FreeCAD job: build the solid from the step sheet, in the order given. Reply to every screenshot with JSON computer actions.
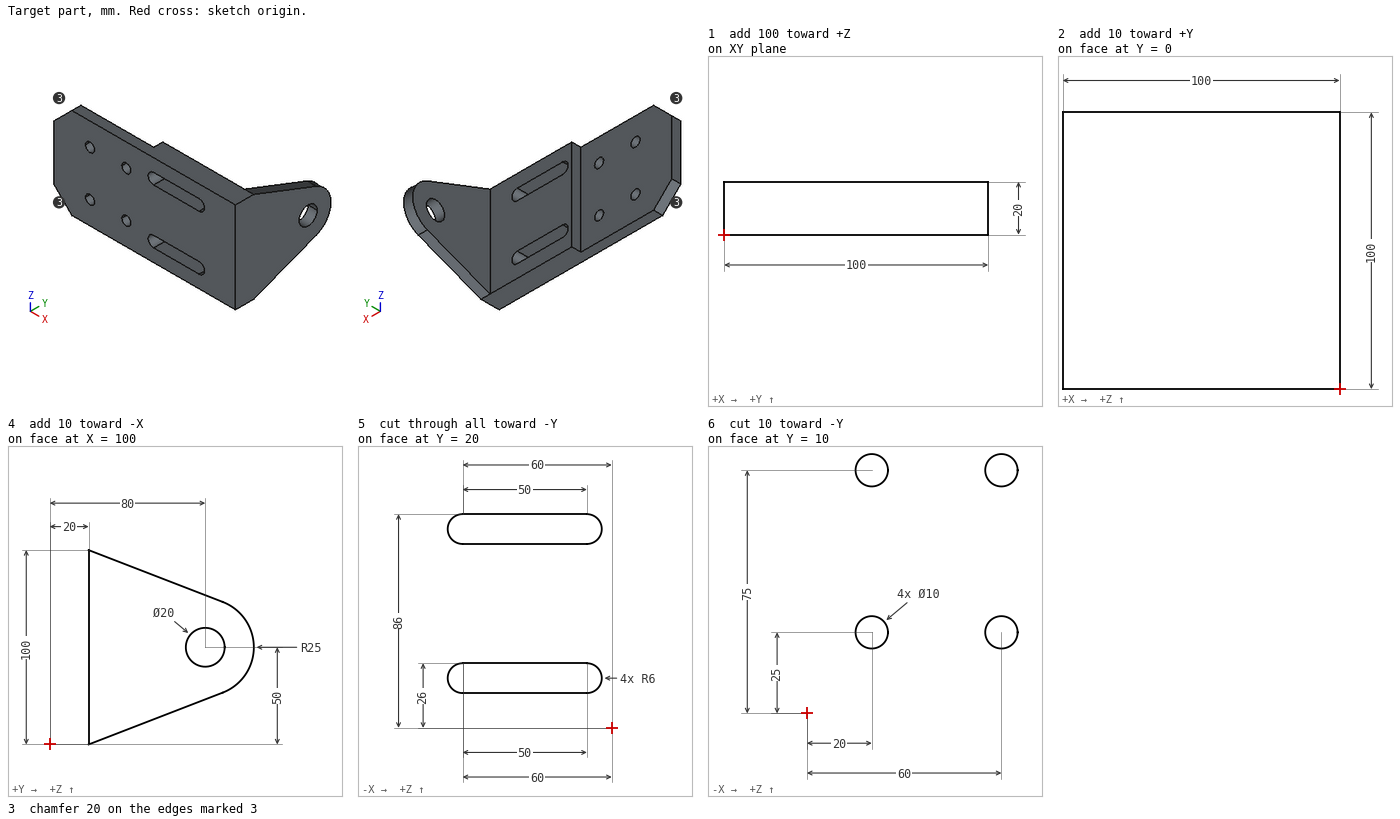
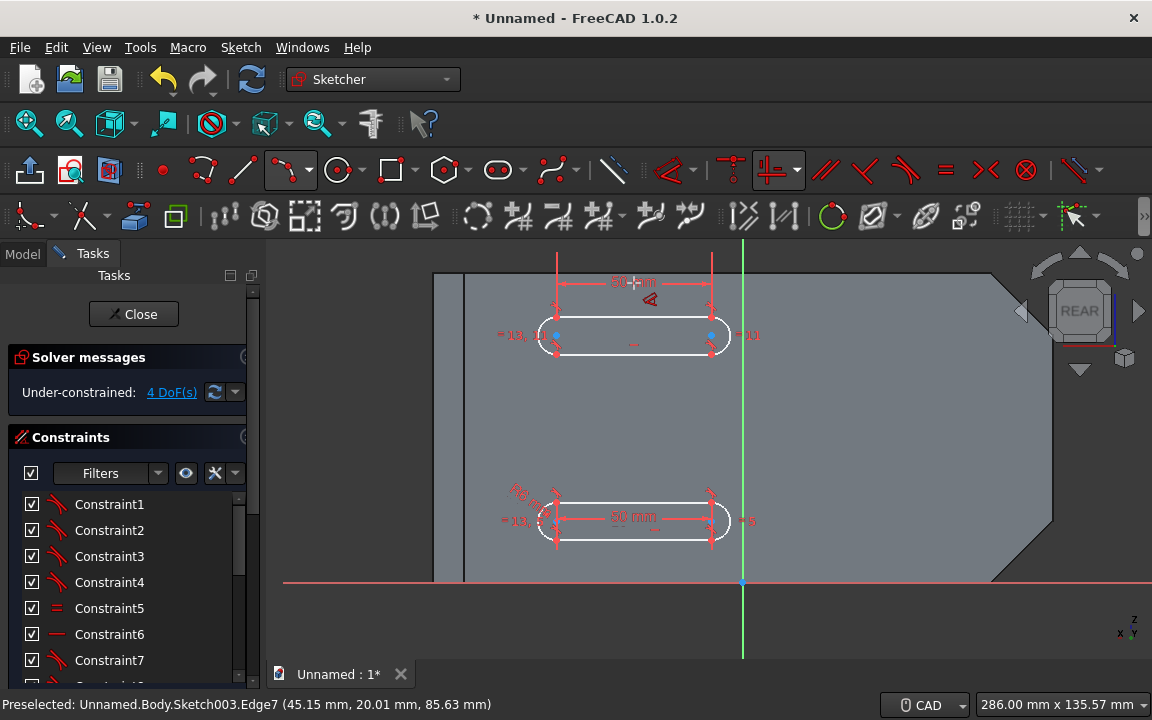
{"action": "left_click", "coordinate": [557, 503]}
{"action": "left_click", "coordinate": [650, 617]}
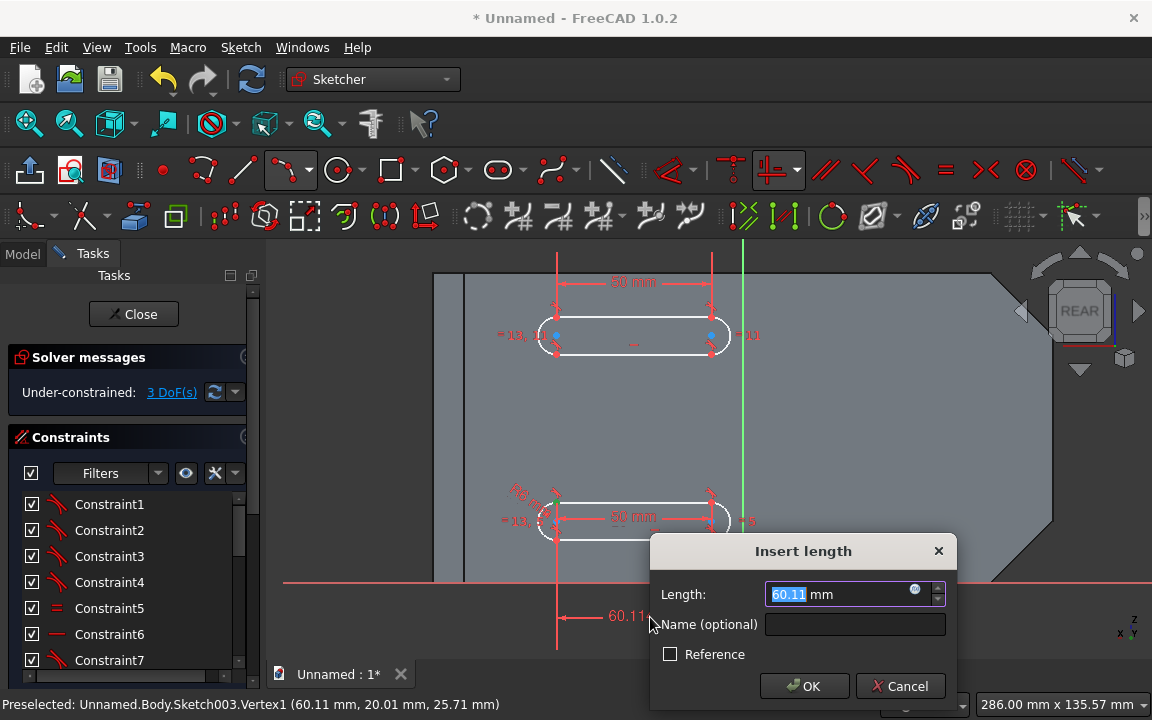
{"action": "type", "text": "60"}
{"action": "key", "text": "Return"}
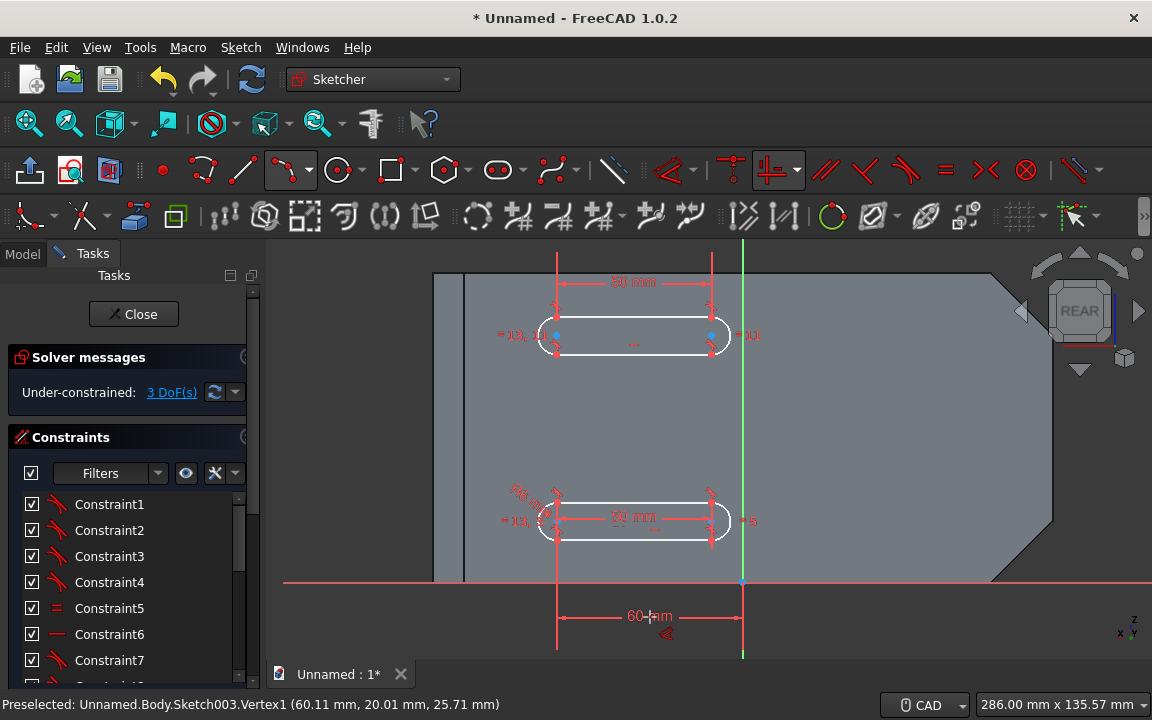
{"action": "left_click", "coordinate": [557, 503]}
{"action": "left_click", "coordinate": [777, 543]}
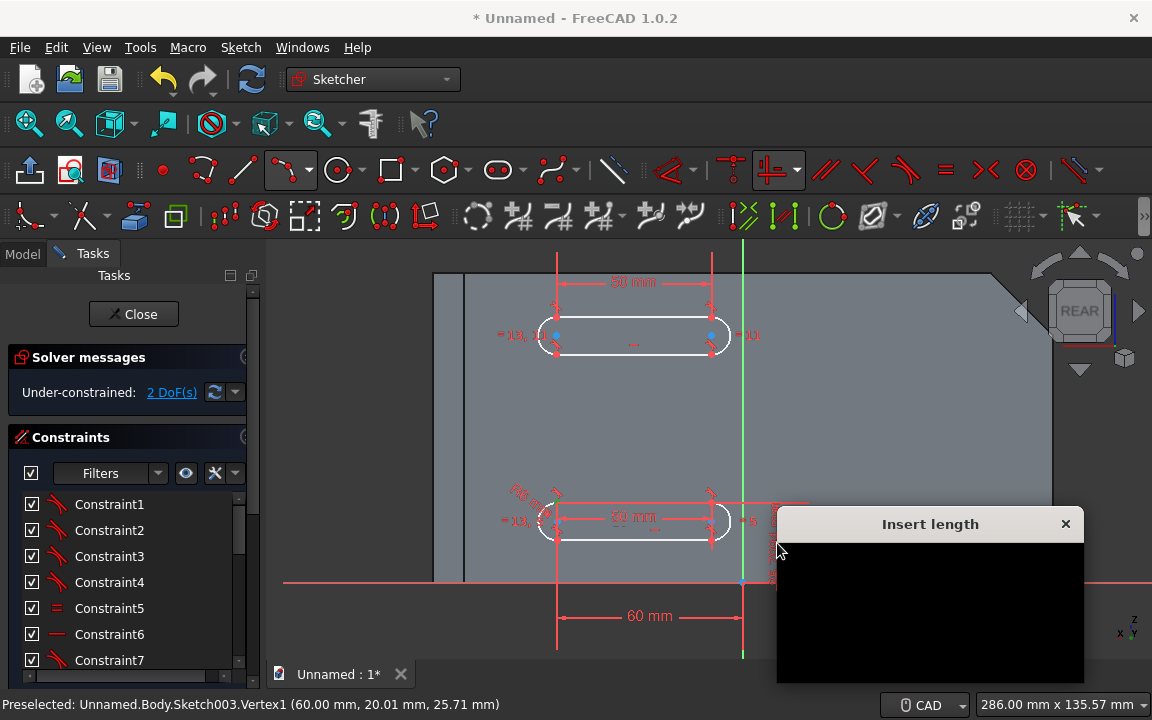
{"action": "type", "text": "26"}
{"action": "key", "text": "Return"}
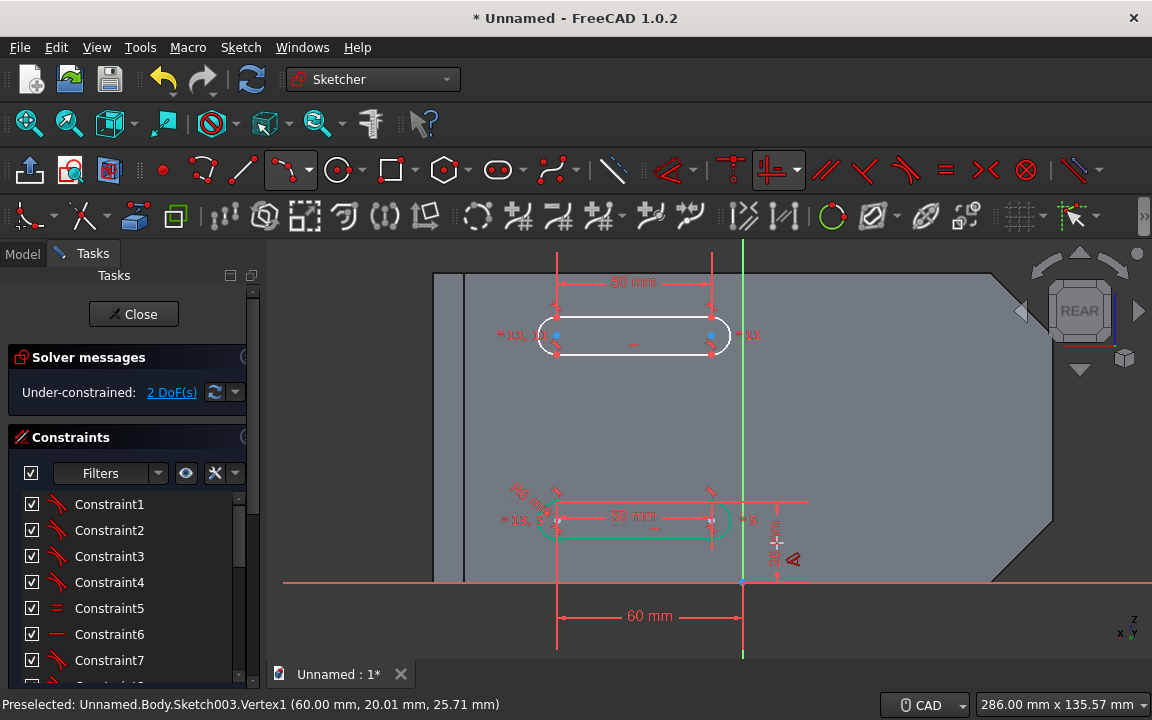
{"action": "left_click", "coordinate": [557, 317]}
{"action": "left_click", "coordinate": [715, 283]}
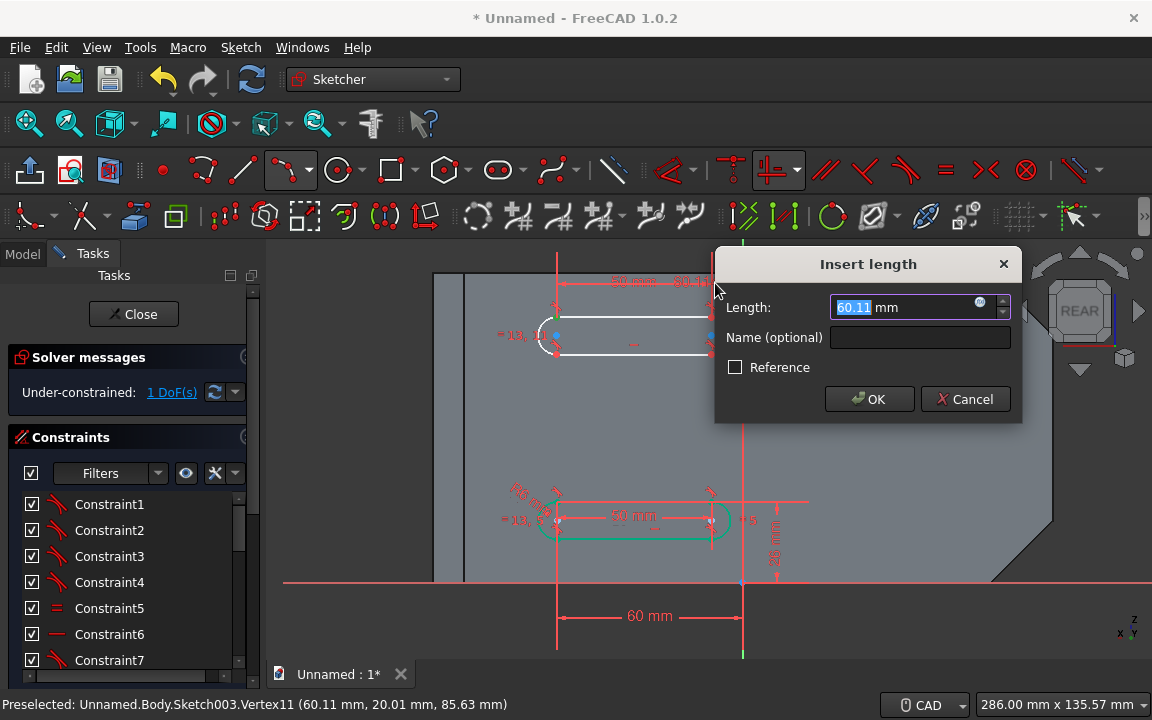
{"action": "type", "text": "60"}
{"action": "key", "text": "Return"}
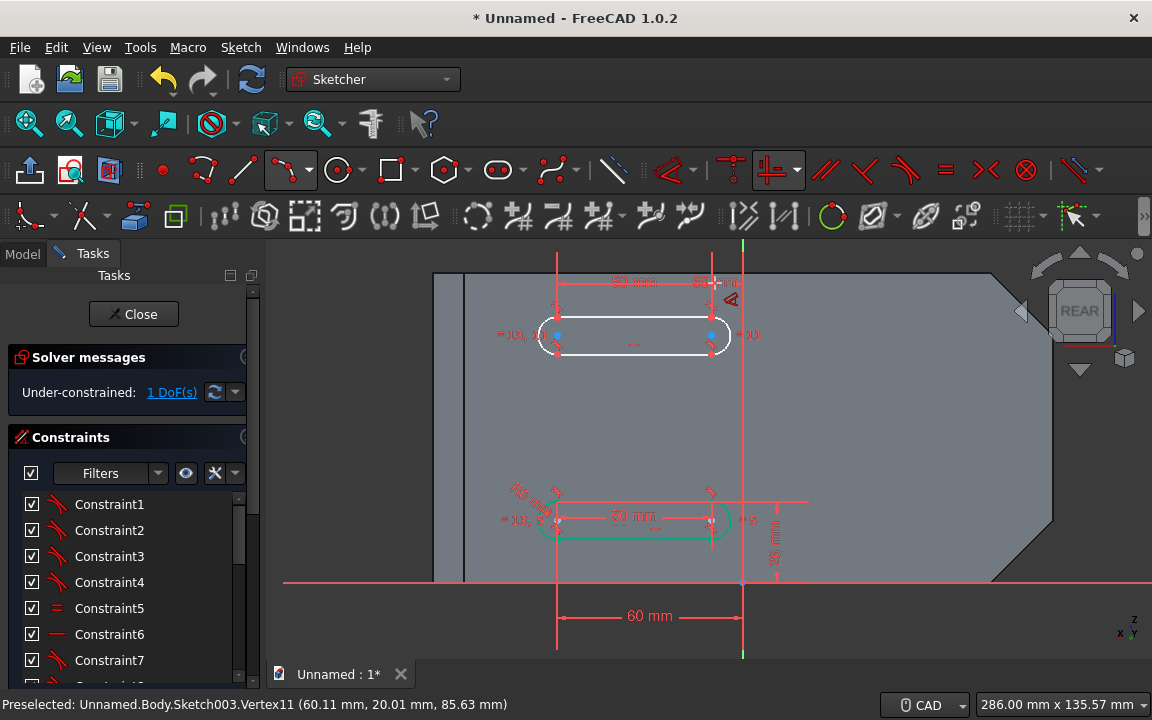
{"action": "left_click", "coordinate": [557, 317]}
{"action": "left_click", "coordinate": [777, 450]}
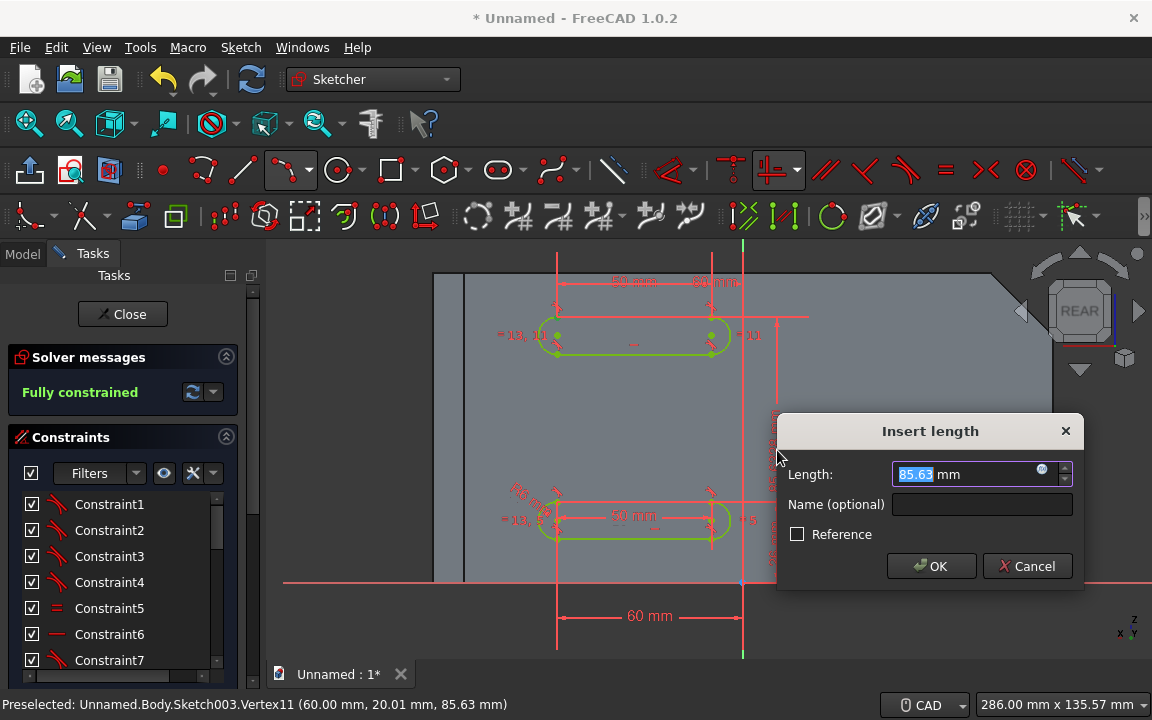
{"action": "type", "text": "86"}
{"action": "key", "text": "Return"}
{"action": "key", "text": "Escape"}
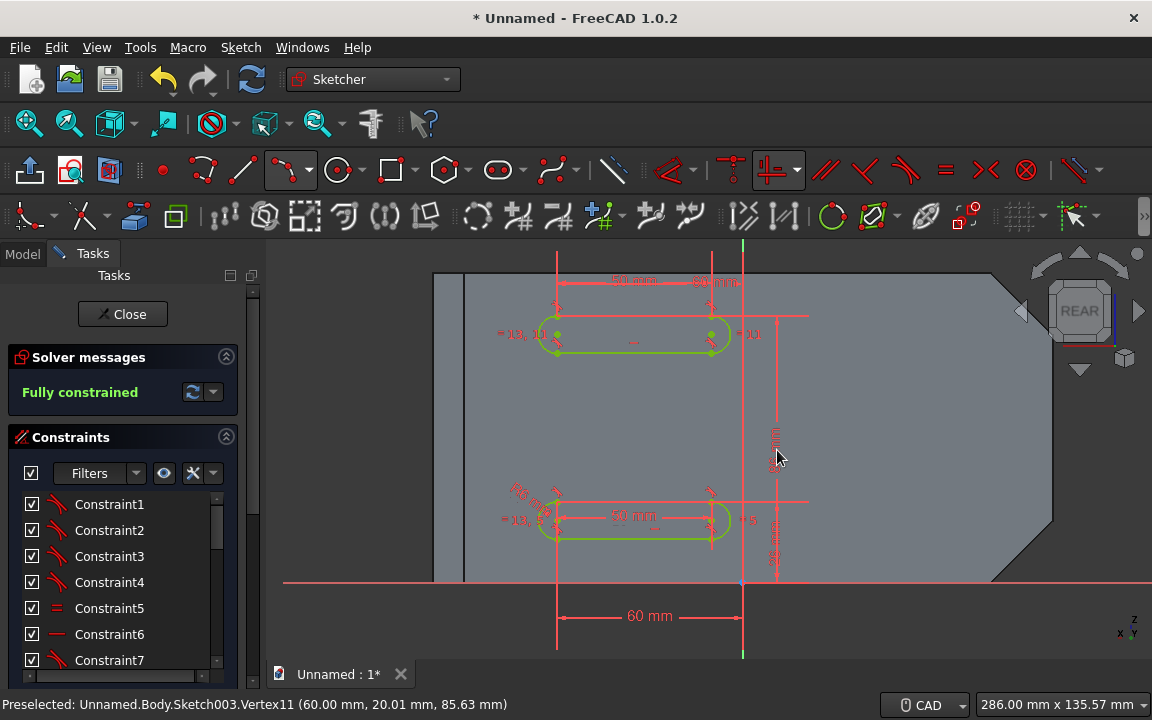
{"action": "left_click", "coordinate": [123, 314]}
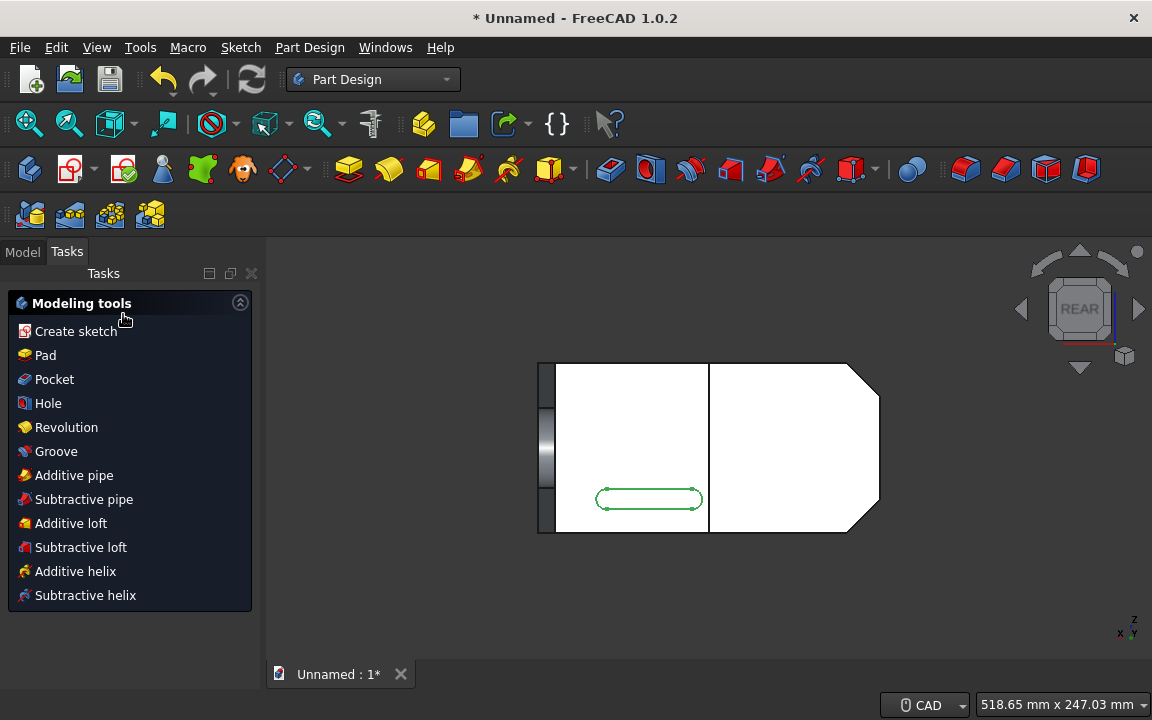
{"action": "left_click", "coordinate": [612, 170]}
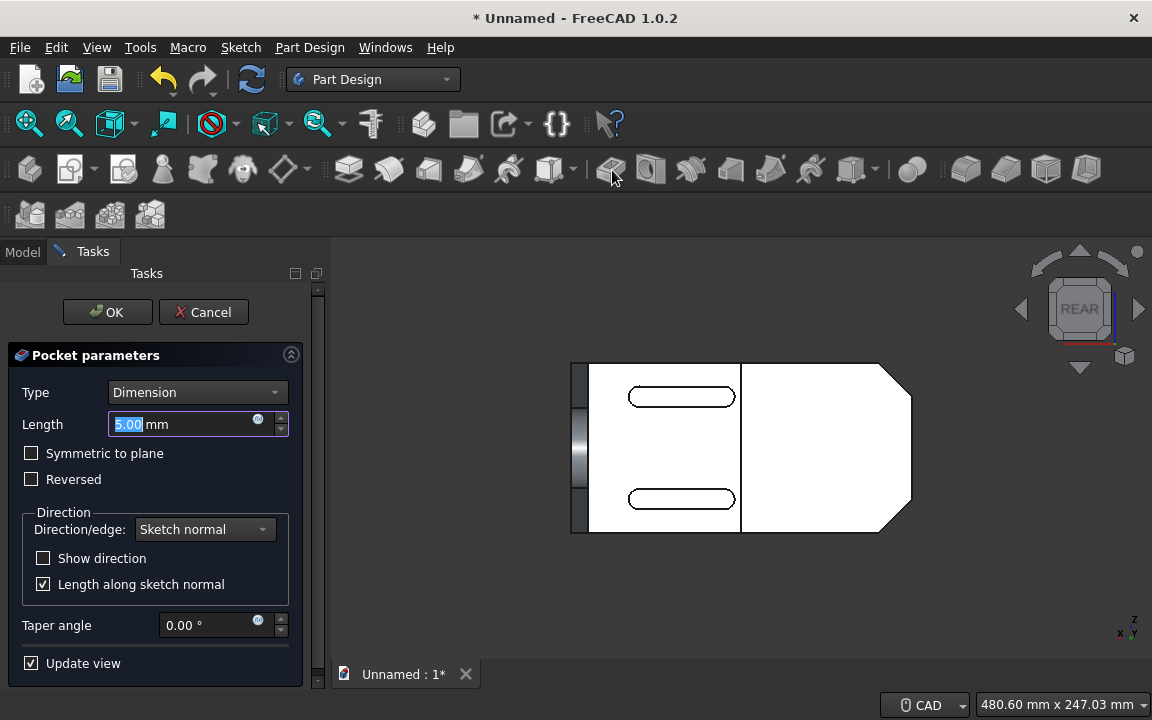
{"action": "left_click", "coordinate": [198, 392]}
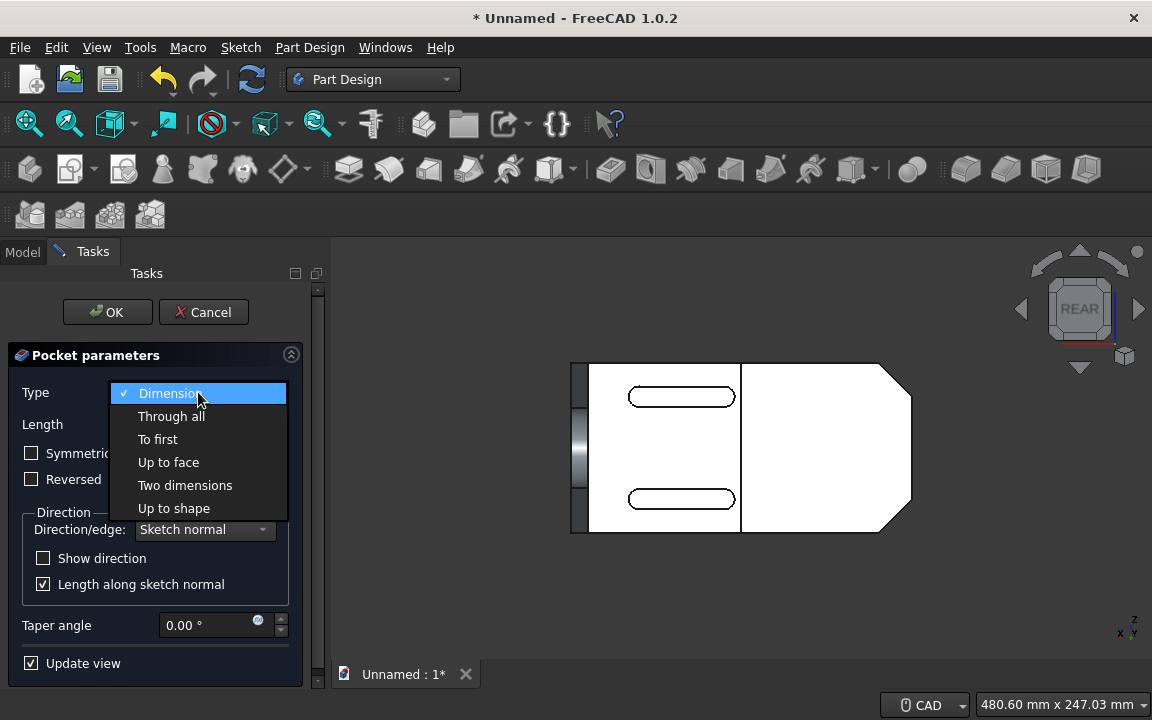
{"action": "left_click", "coordinate": [198, 416]}